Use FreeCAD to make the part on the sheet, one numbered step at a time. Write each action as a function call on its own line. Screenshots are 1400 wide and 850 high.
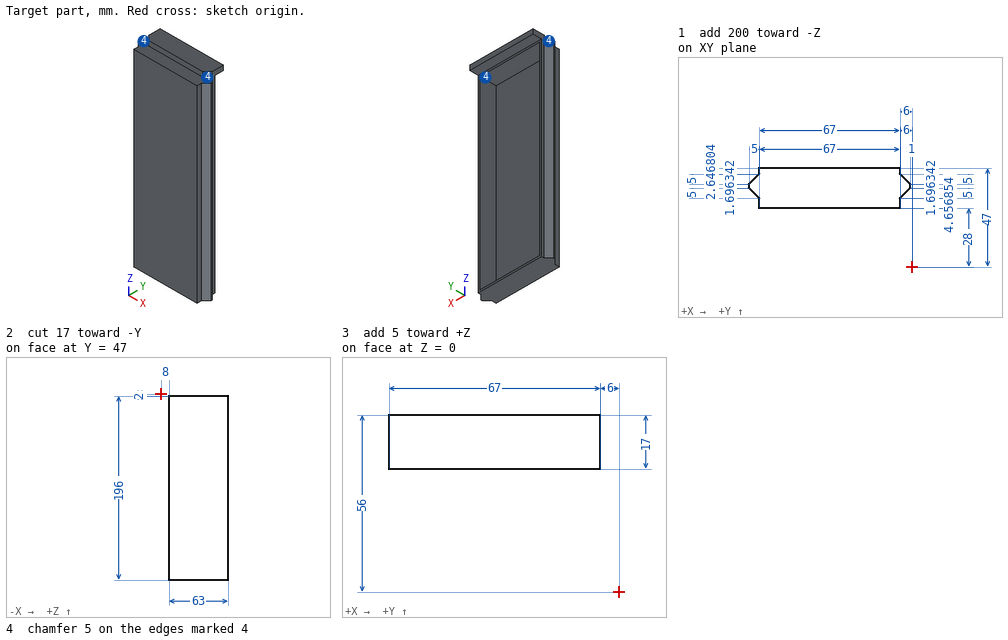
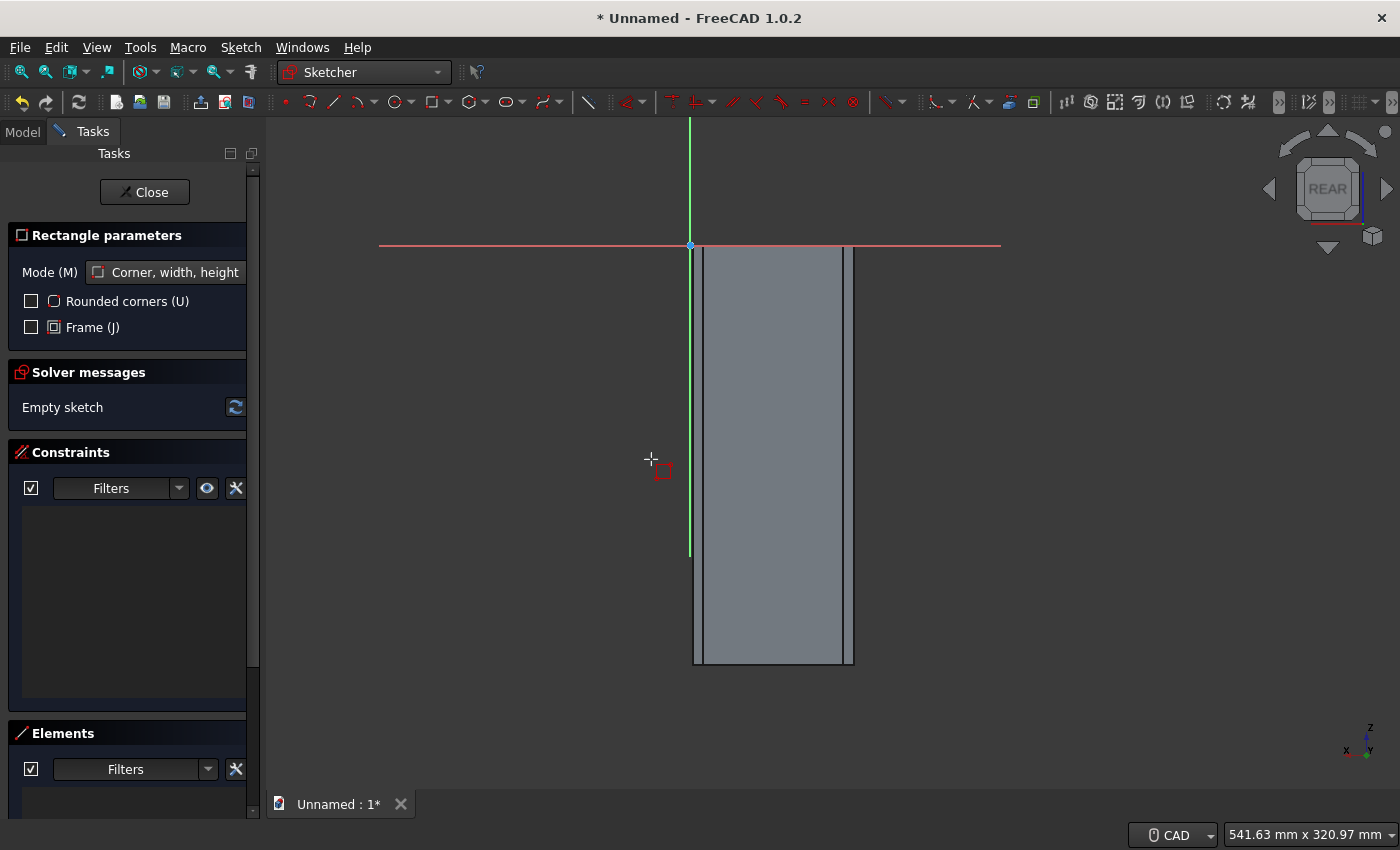
scroll(707, 250, up, 7)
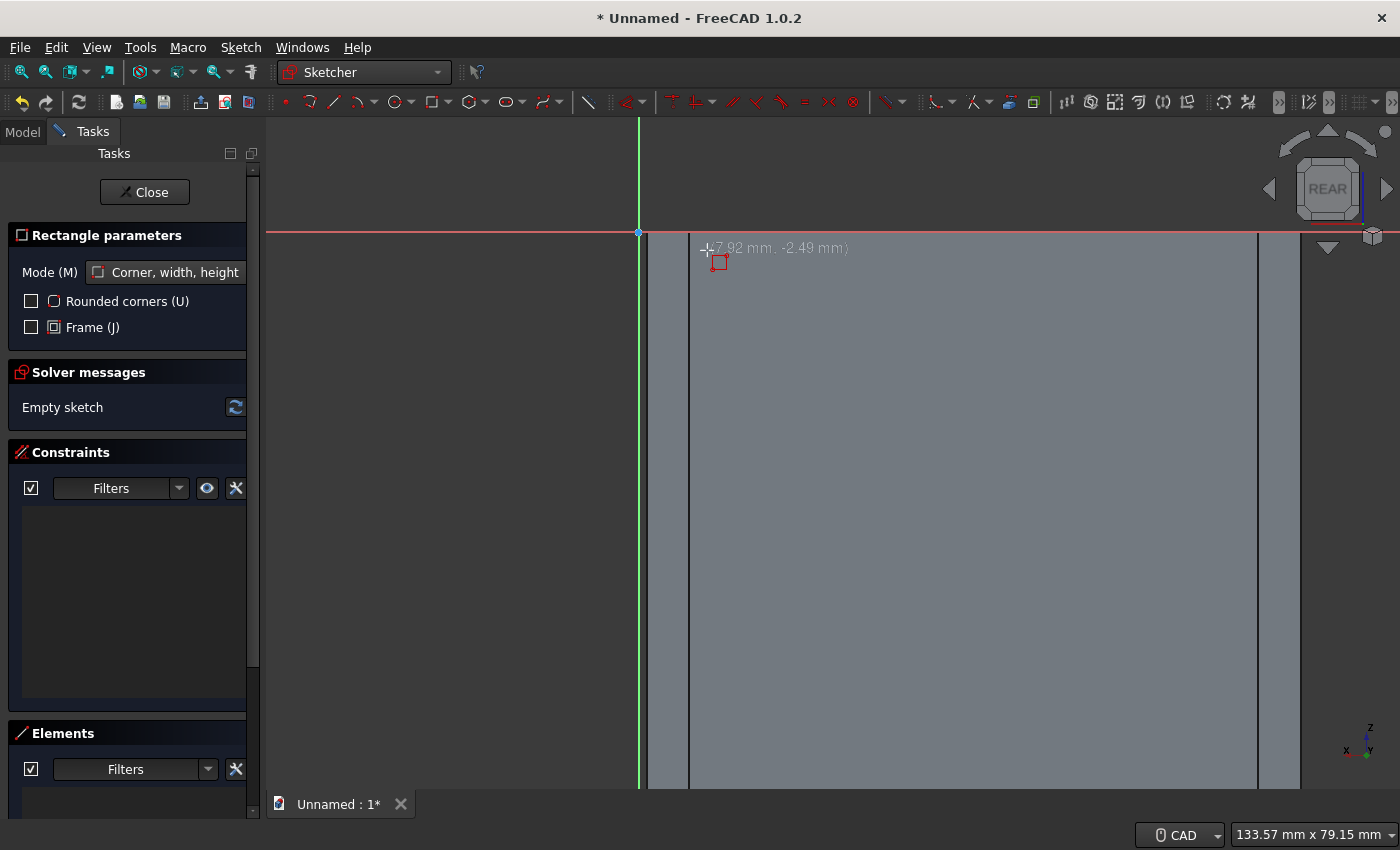
click(706, 249)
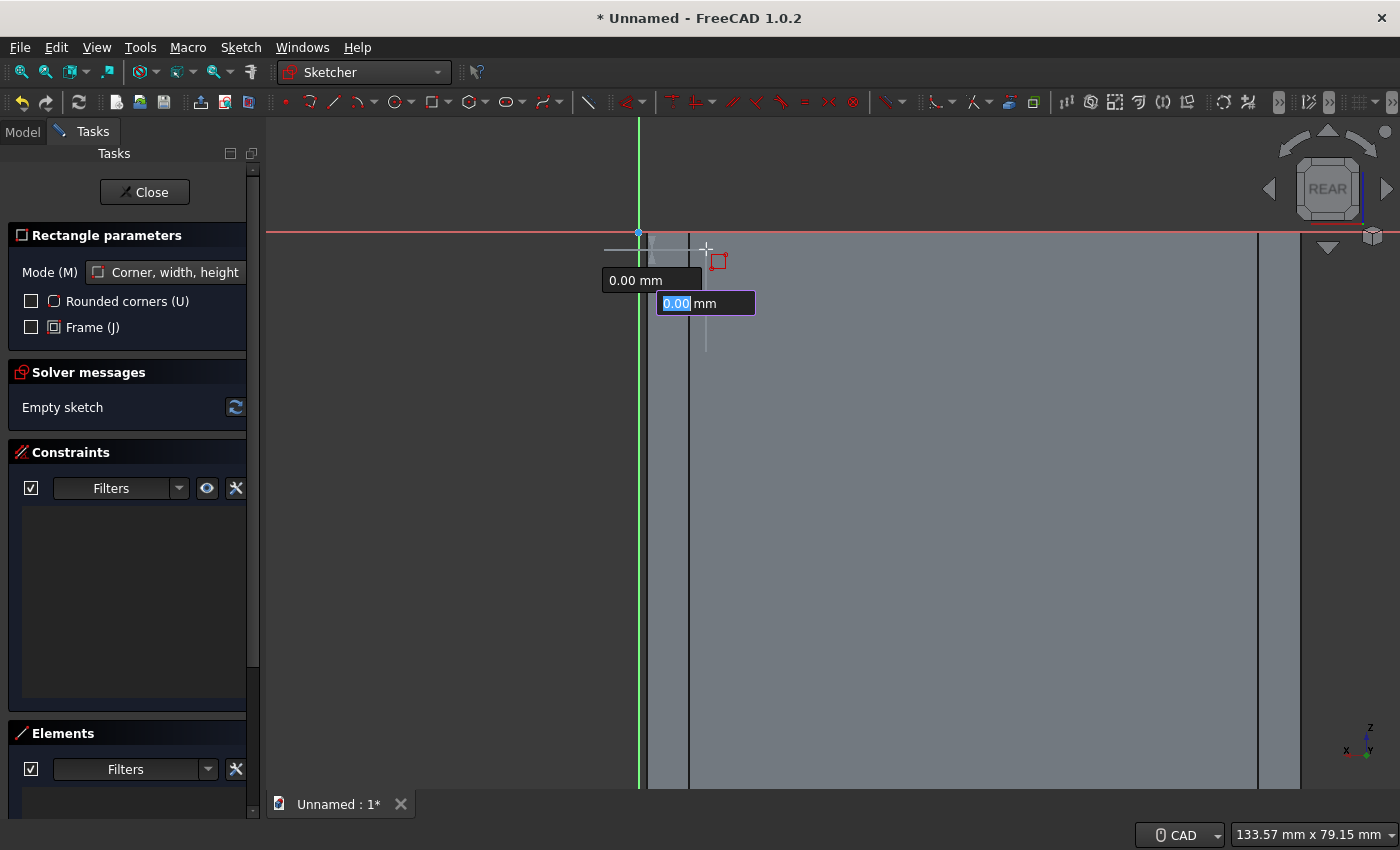
scroll(707, 250, down, 7)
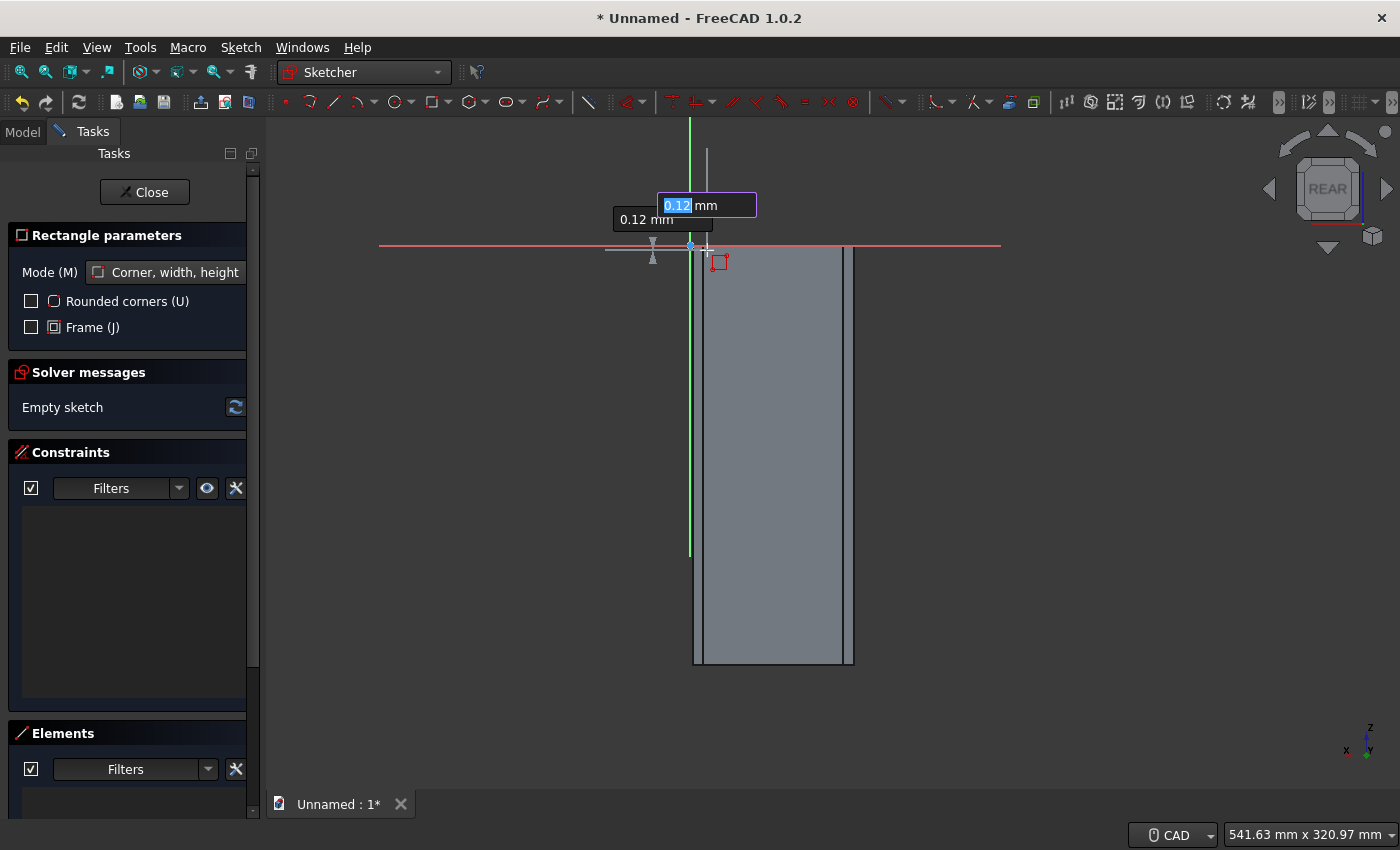
click(839, 660)
key(Escape)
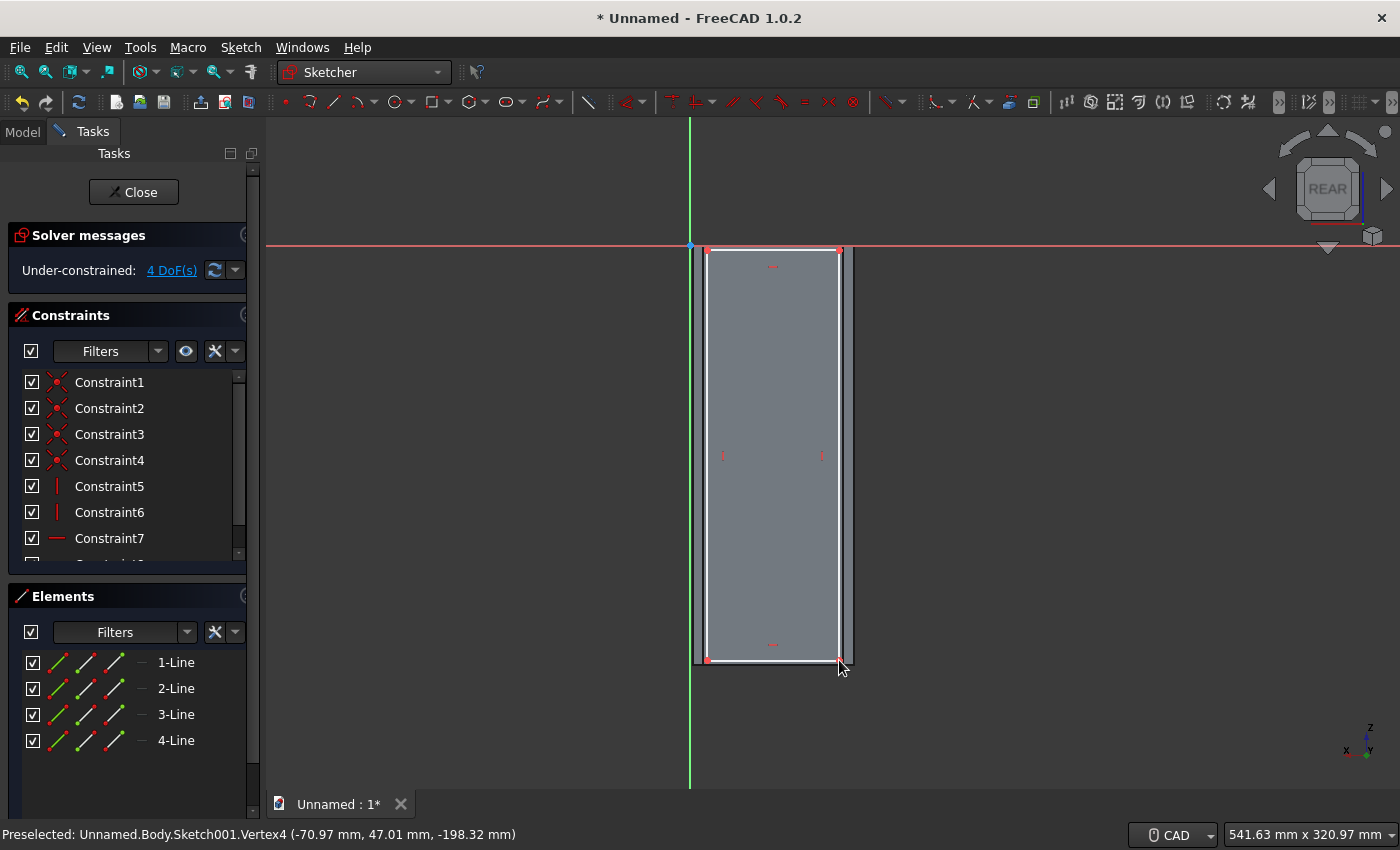
click(626, 102)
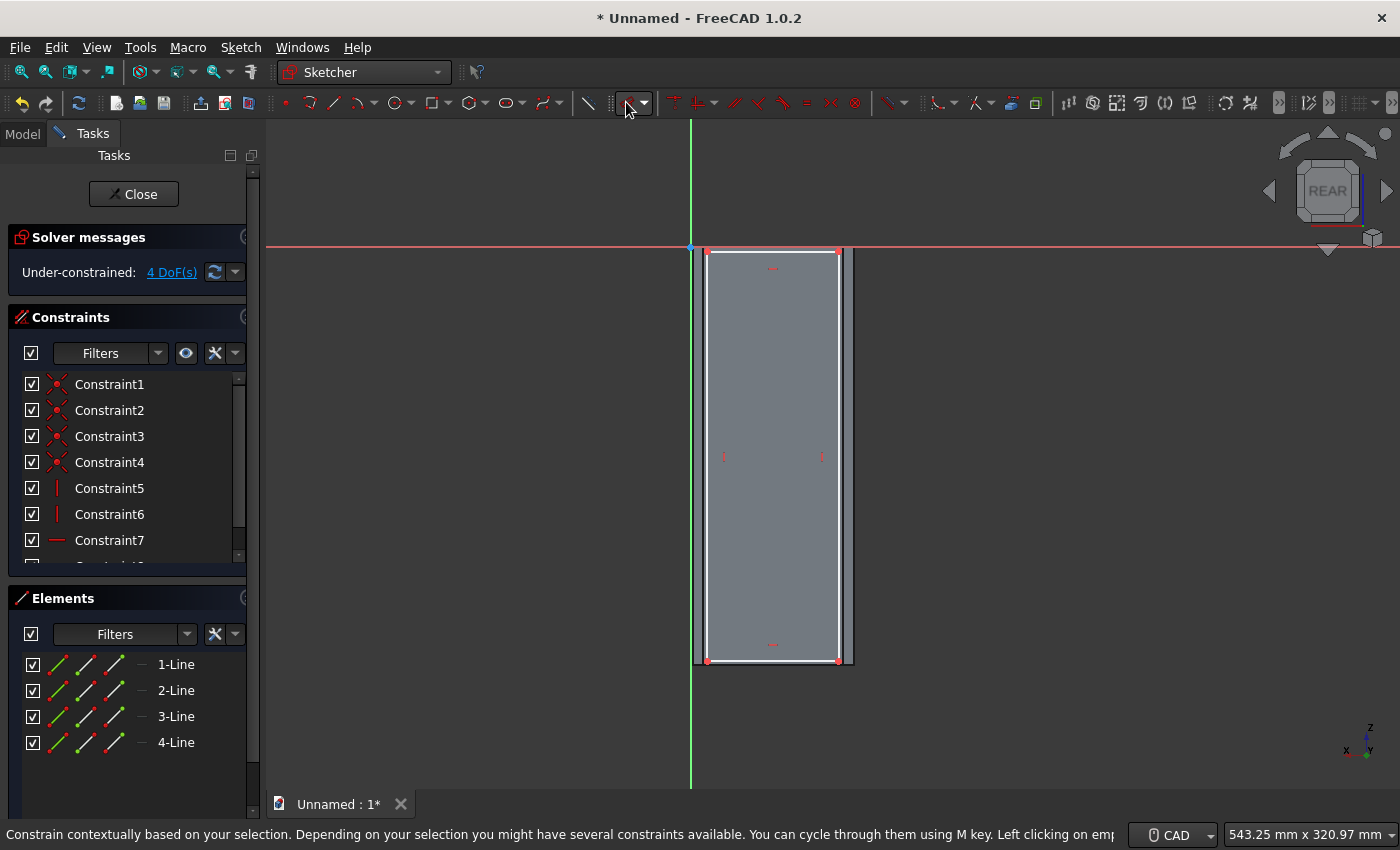
click(747, 661)
click(773, 695)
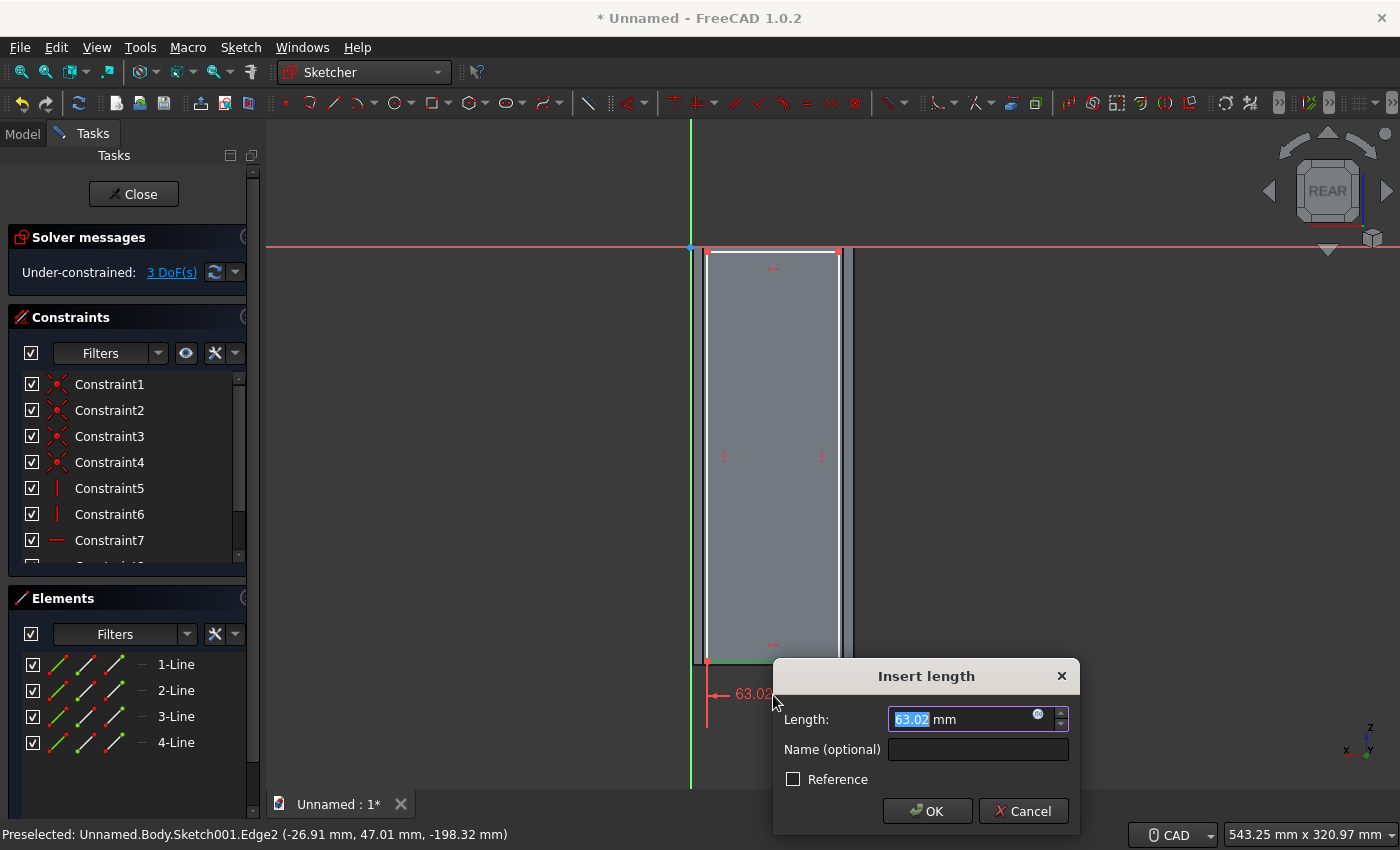
text(63)
key(Return)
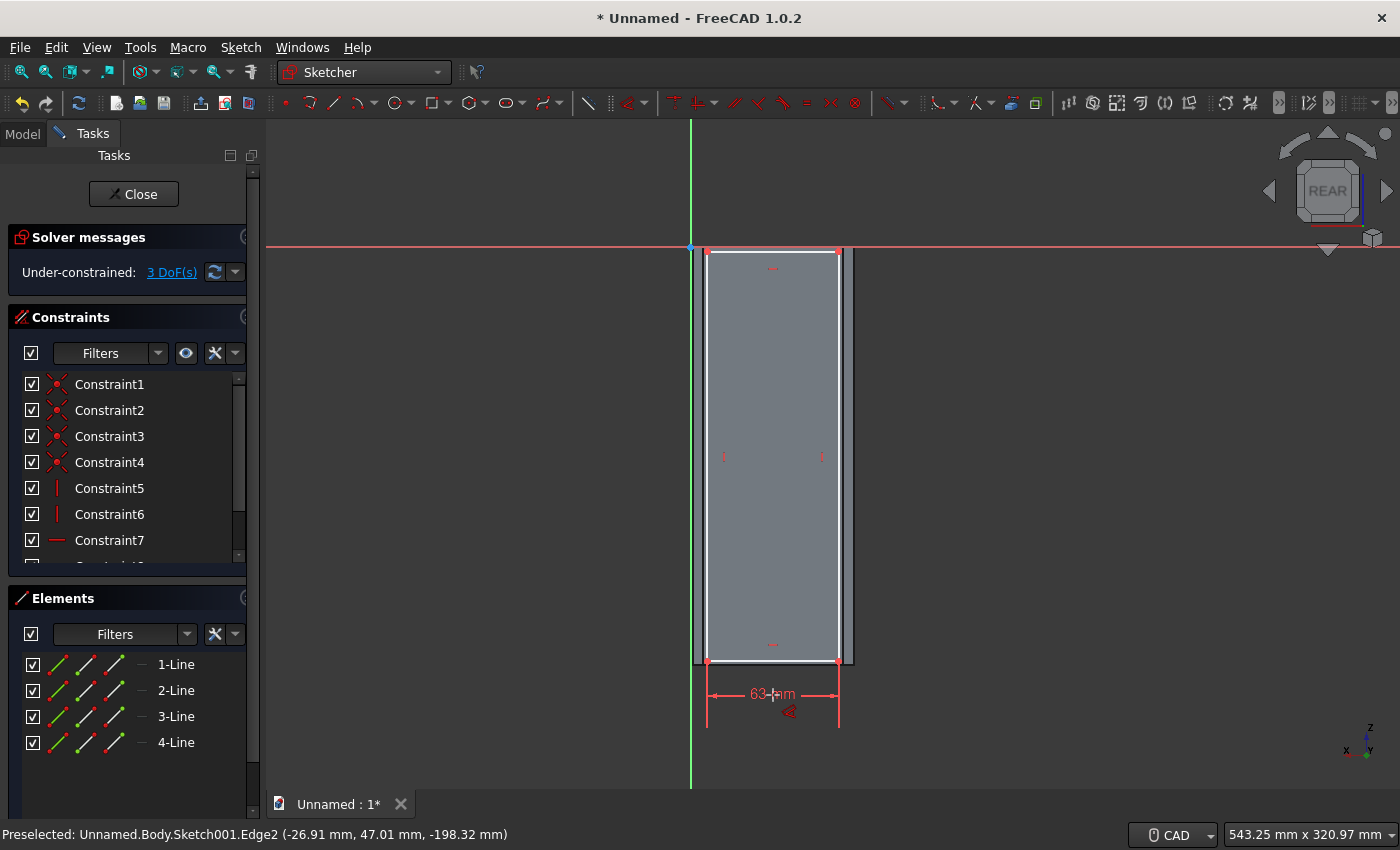
scroll(707, 252, up, 5)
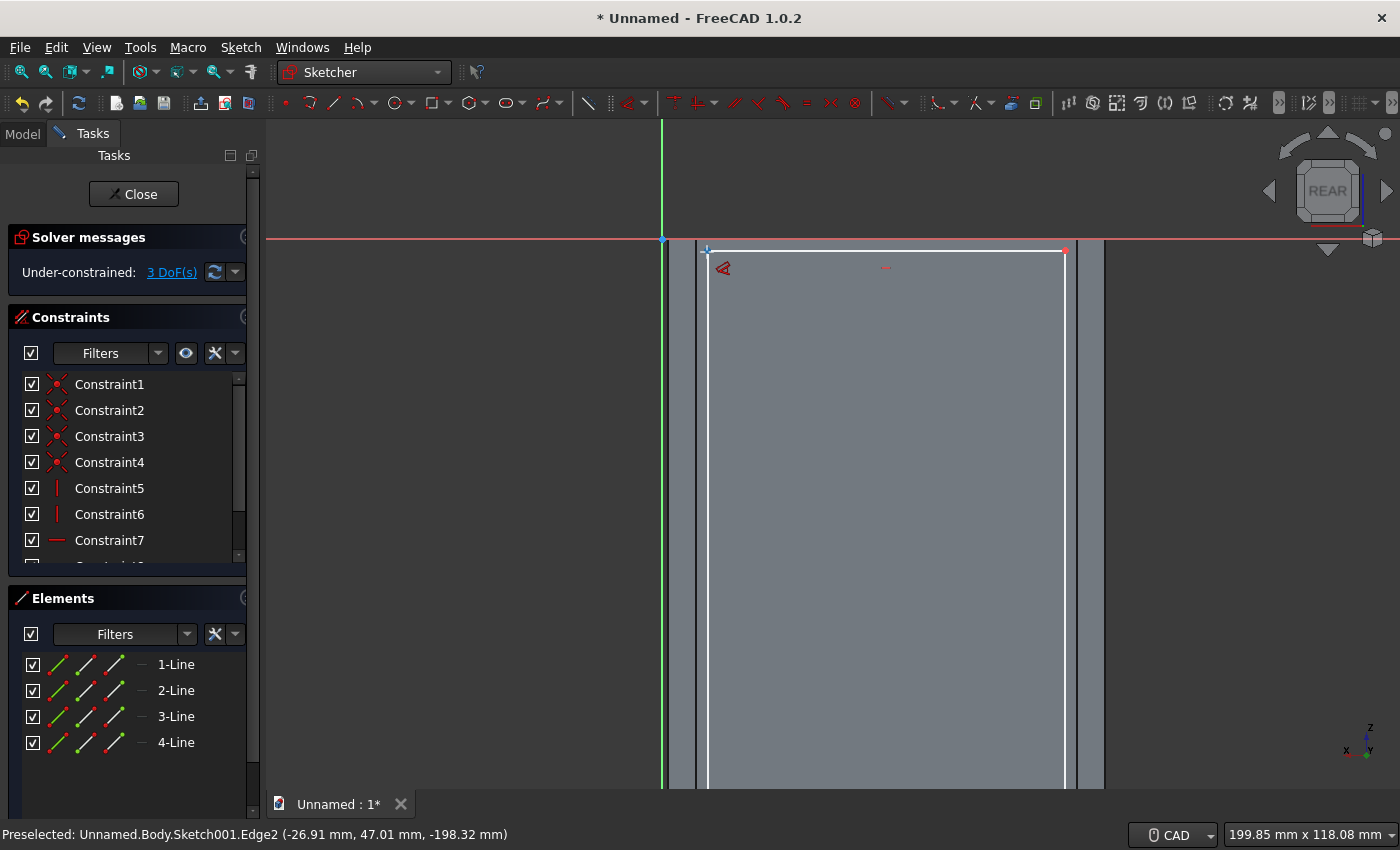
click(708, 251)
click(685, 205)